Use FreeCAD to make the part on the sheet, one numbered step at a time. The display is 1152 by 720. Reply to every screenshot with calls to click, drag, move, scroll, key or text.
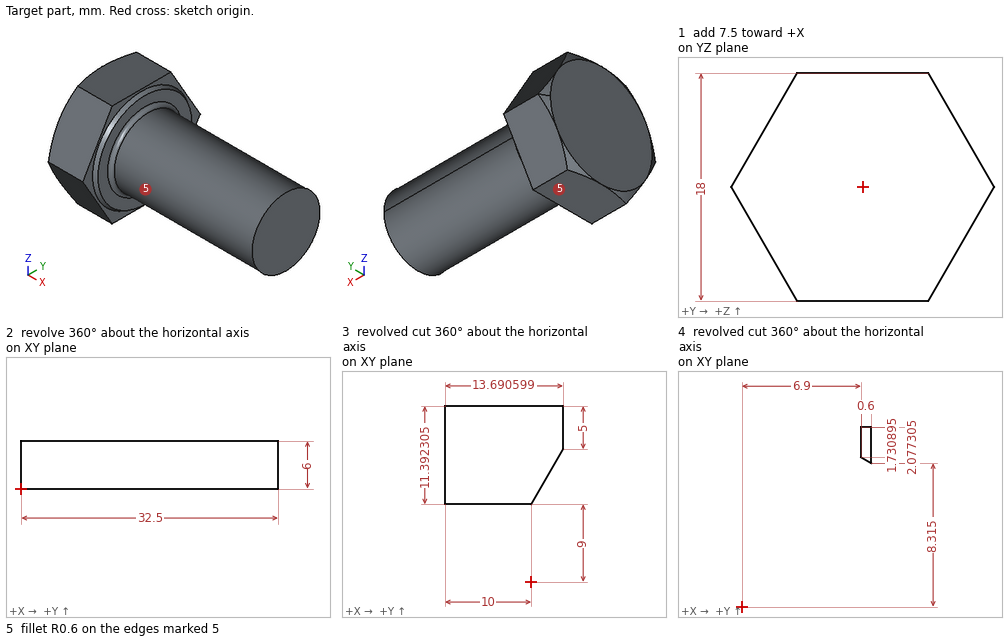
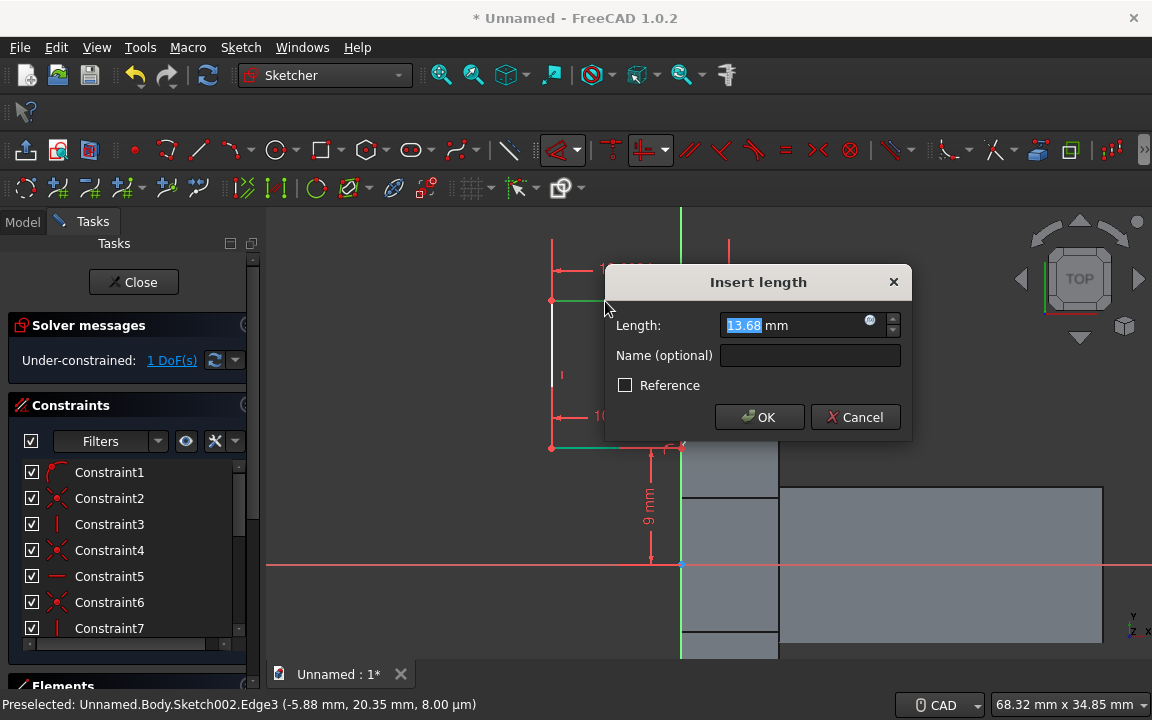
text(13.690599)
key(Return)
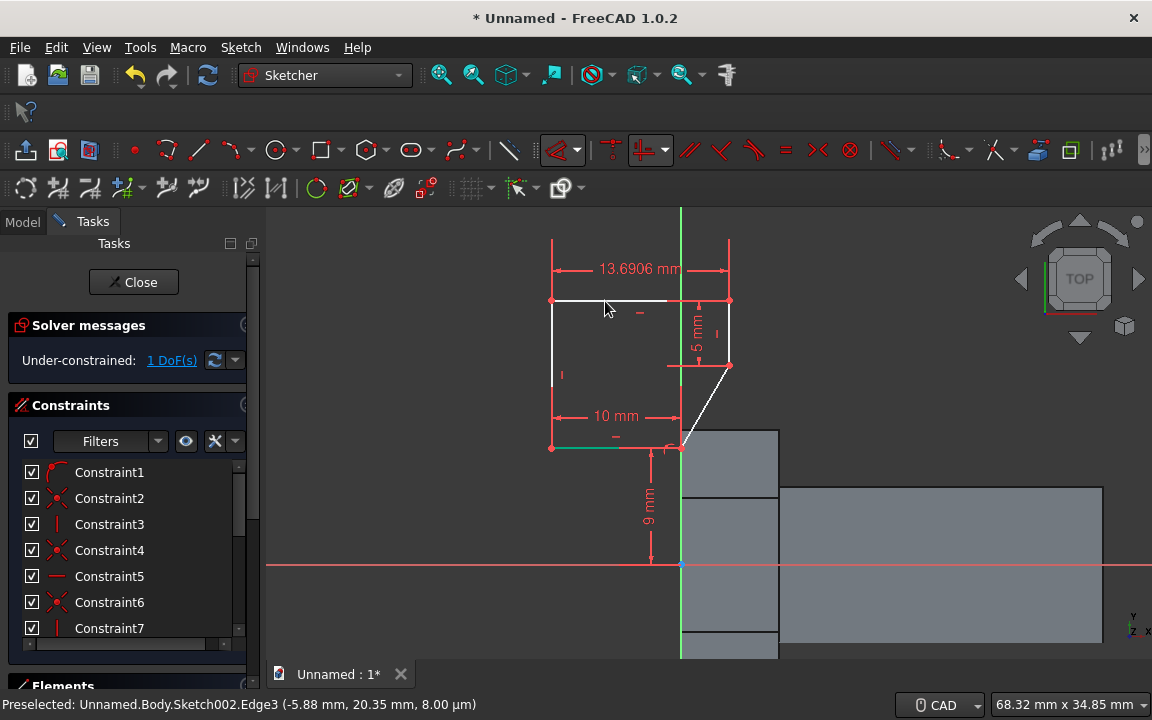
click(552, 345)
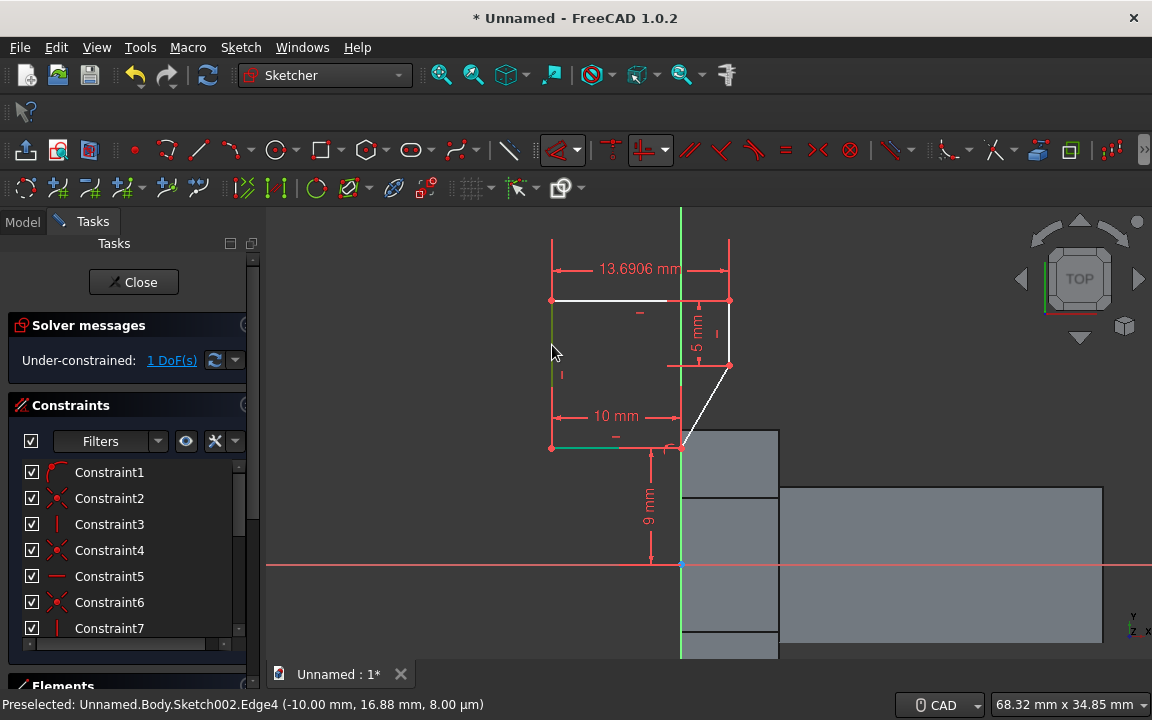
click(580, 150)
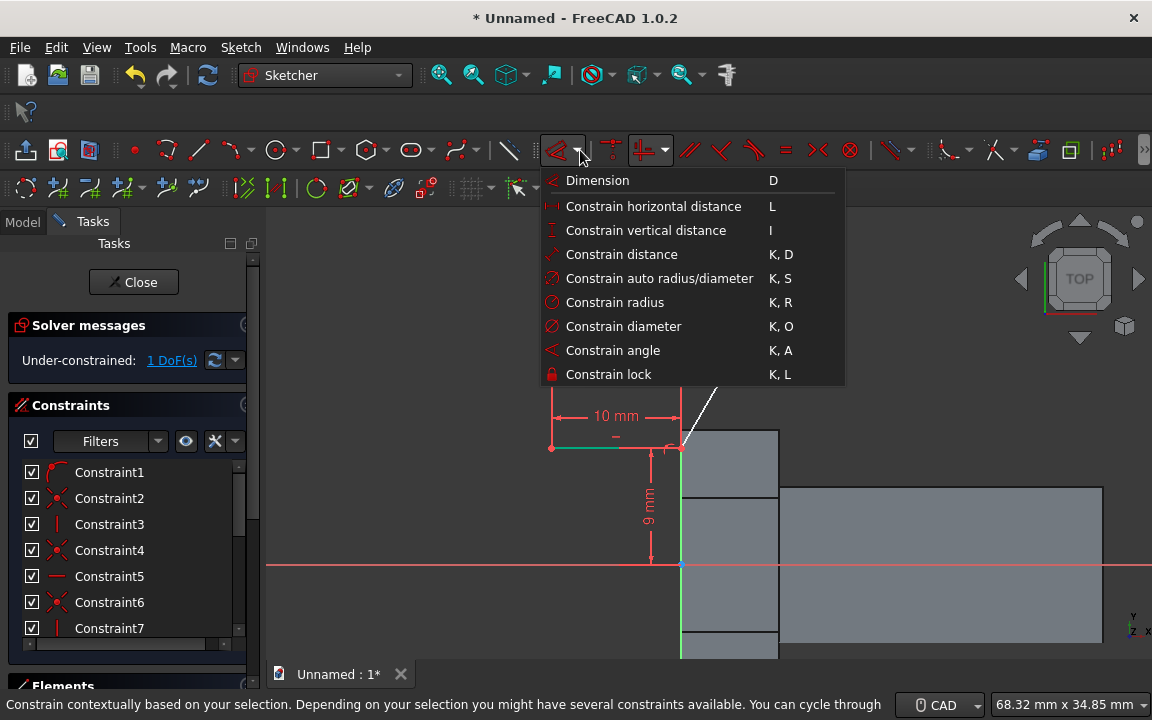
click(693, 230)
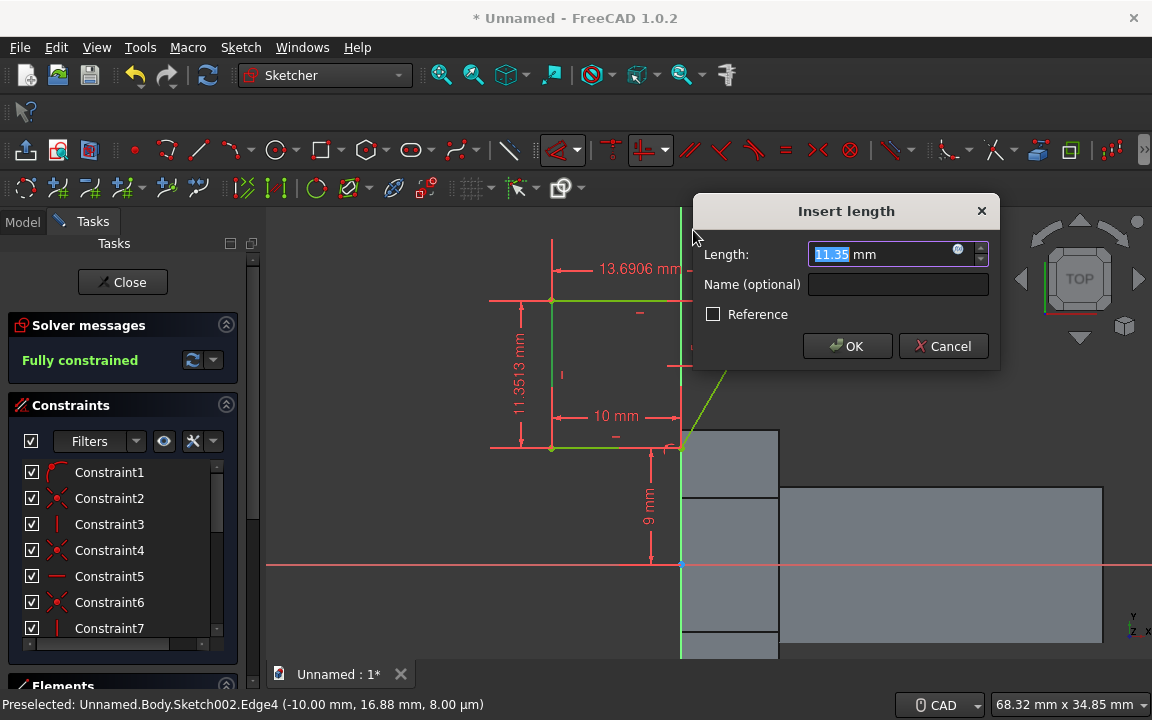
text(11.392305)
key(Return)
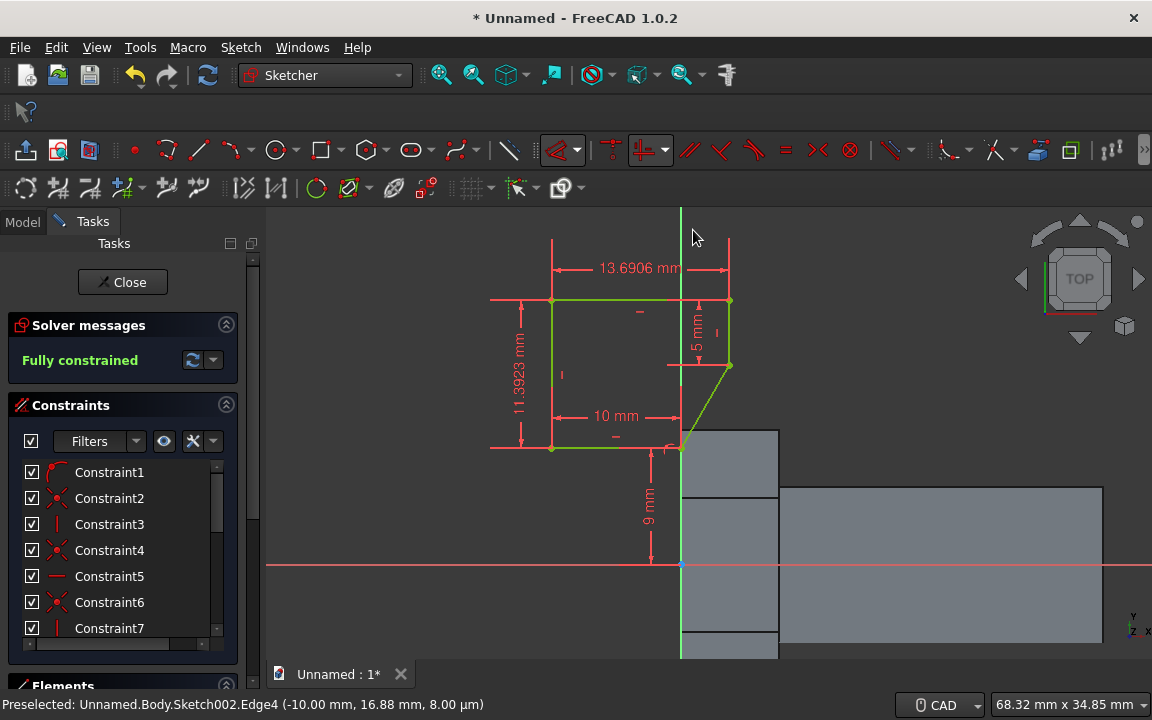
click(123, 282)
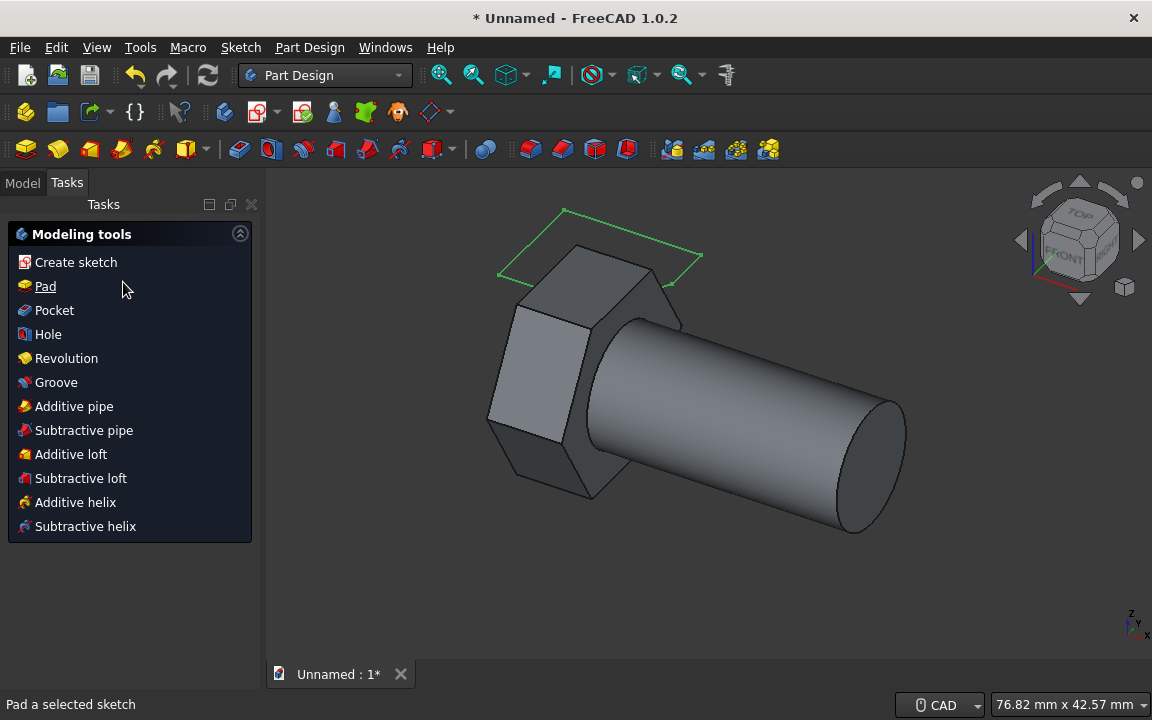
click(304, 150)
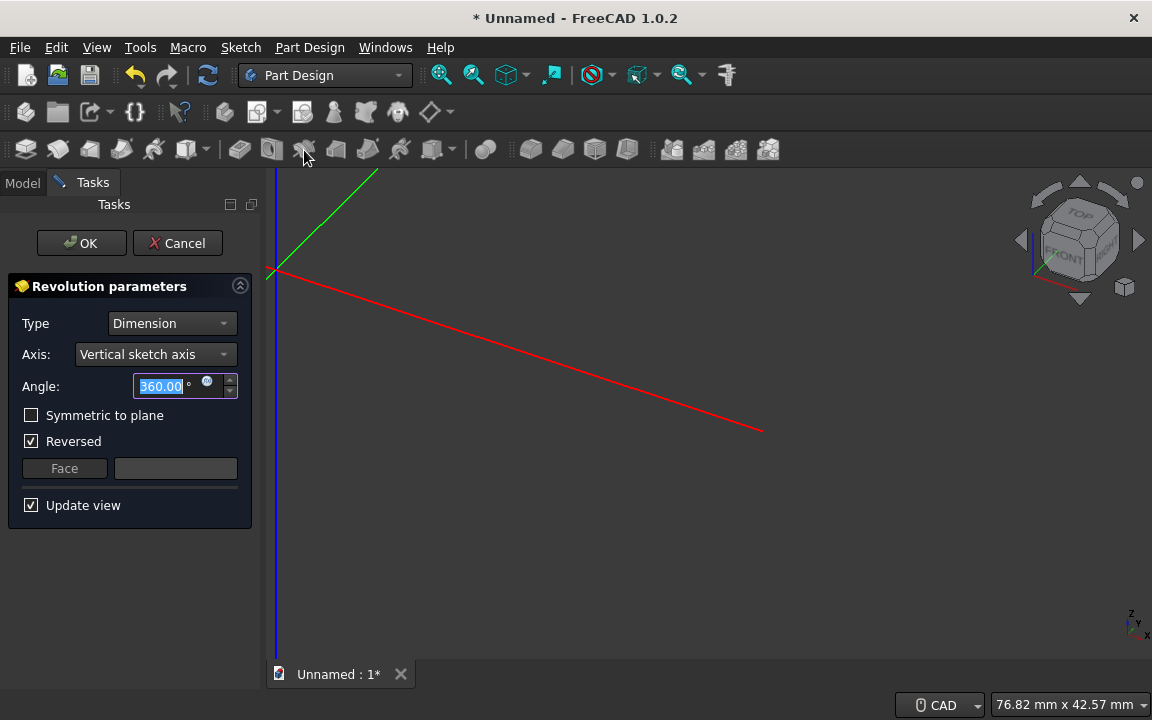
click(156, 354)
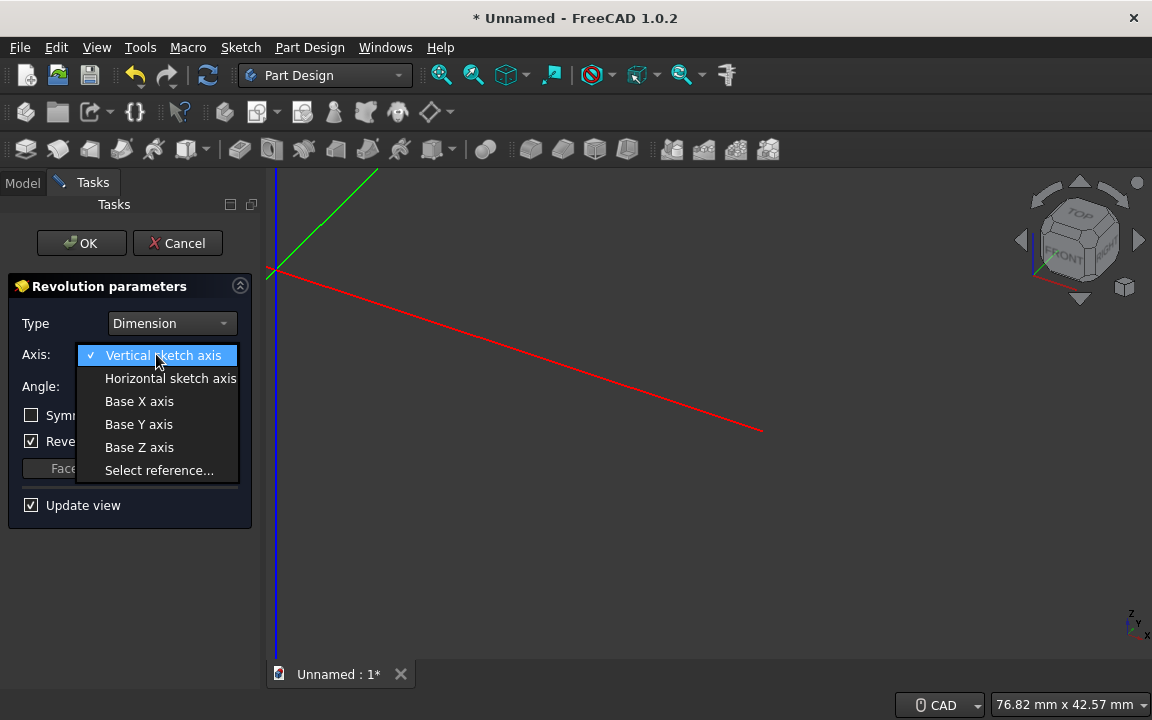
click(156, 378)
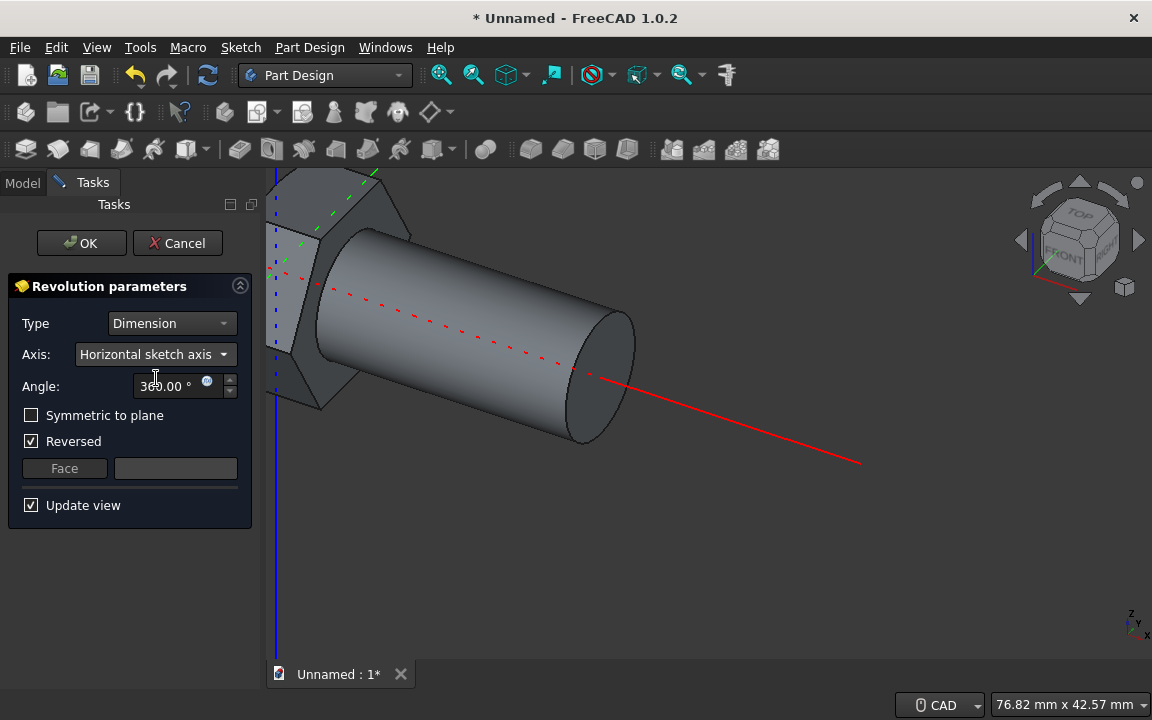
click(82, 243)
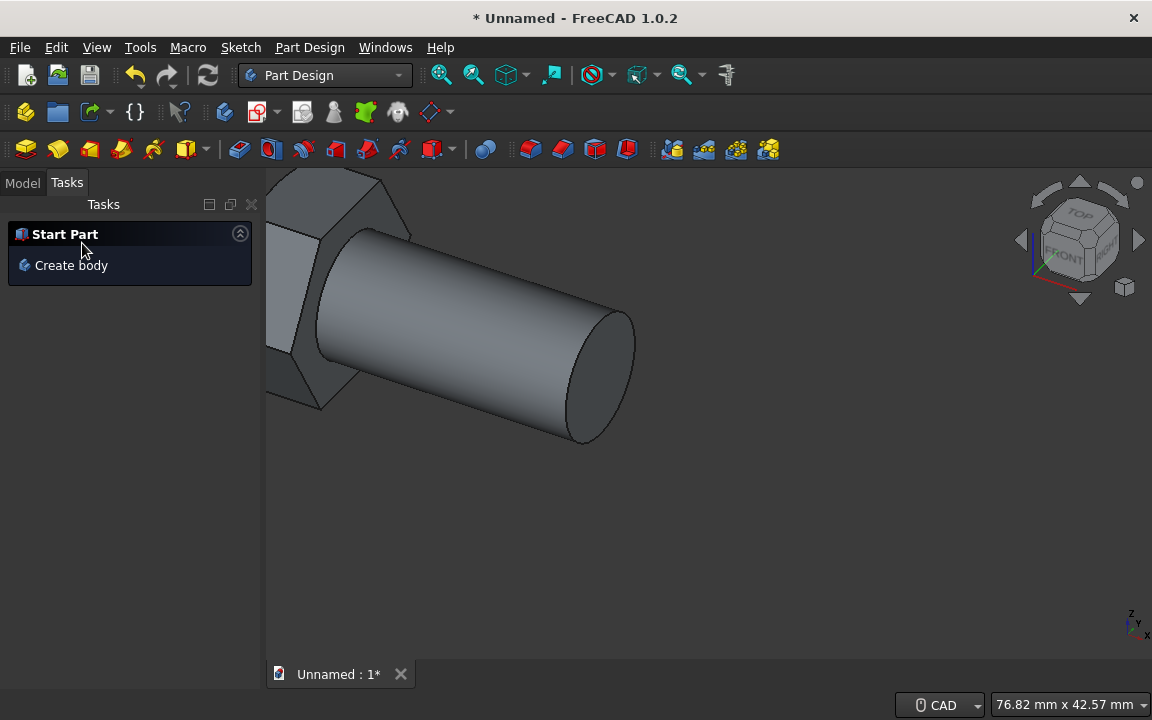
click(442, 76)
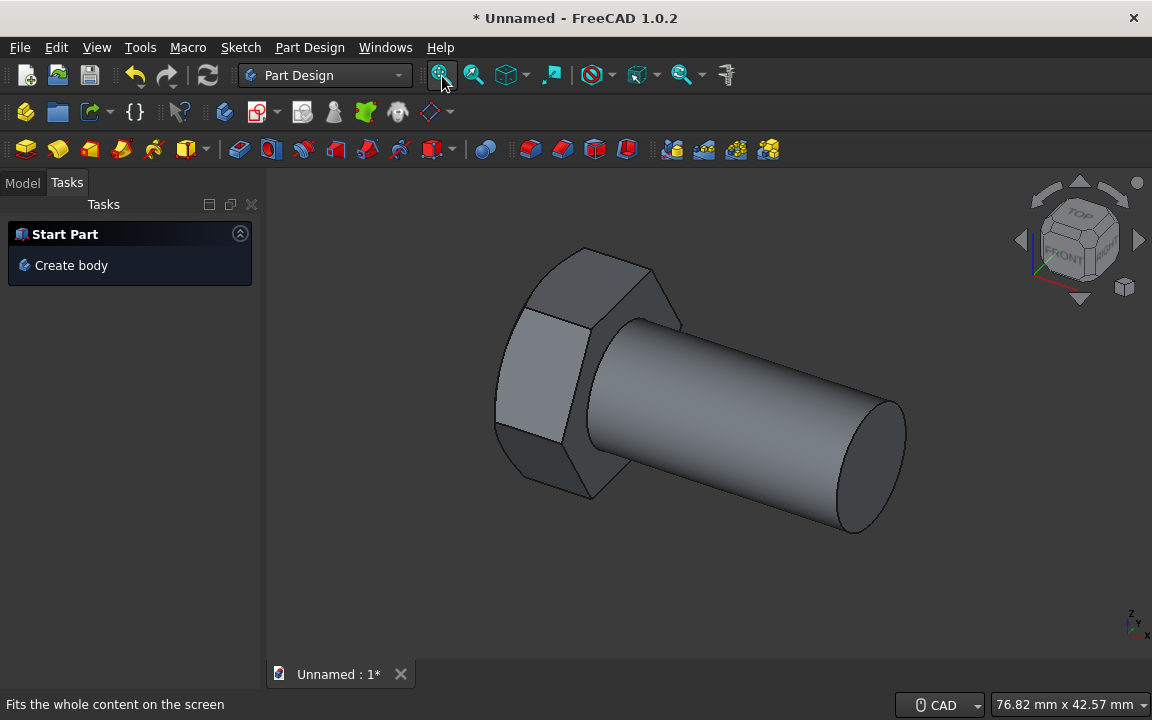
click(258, 112)